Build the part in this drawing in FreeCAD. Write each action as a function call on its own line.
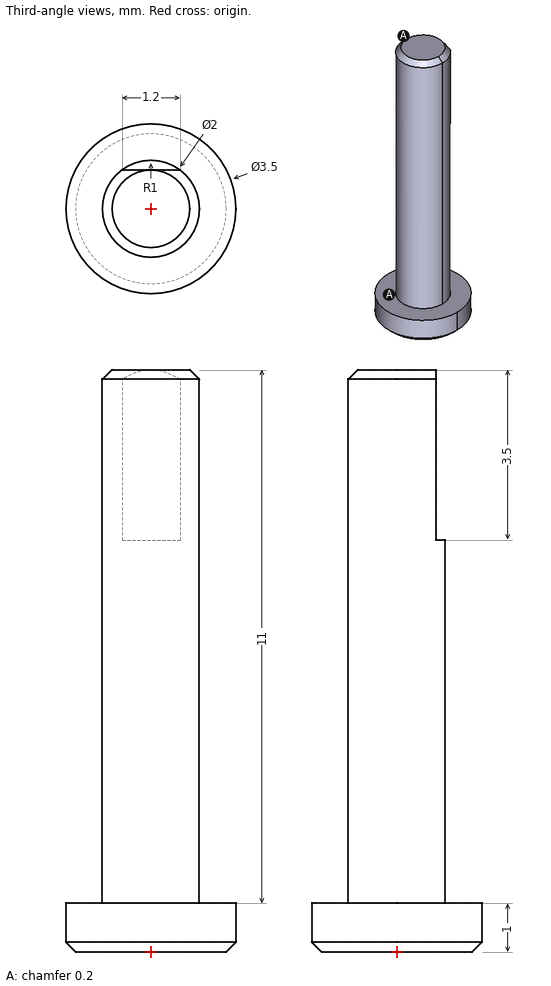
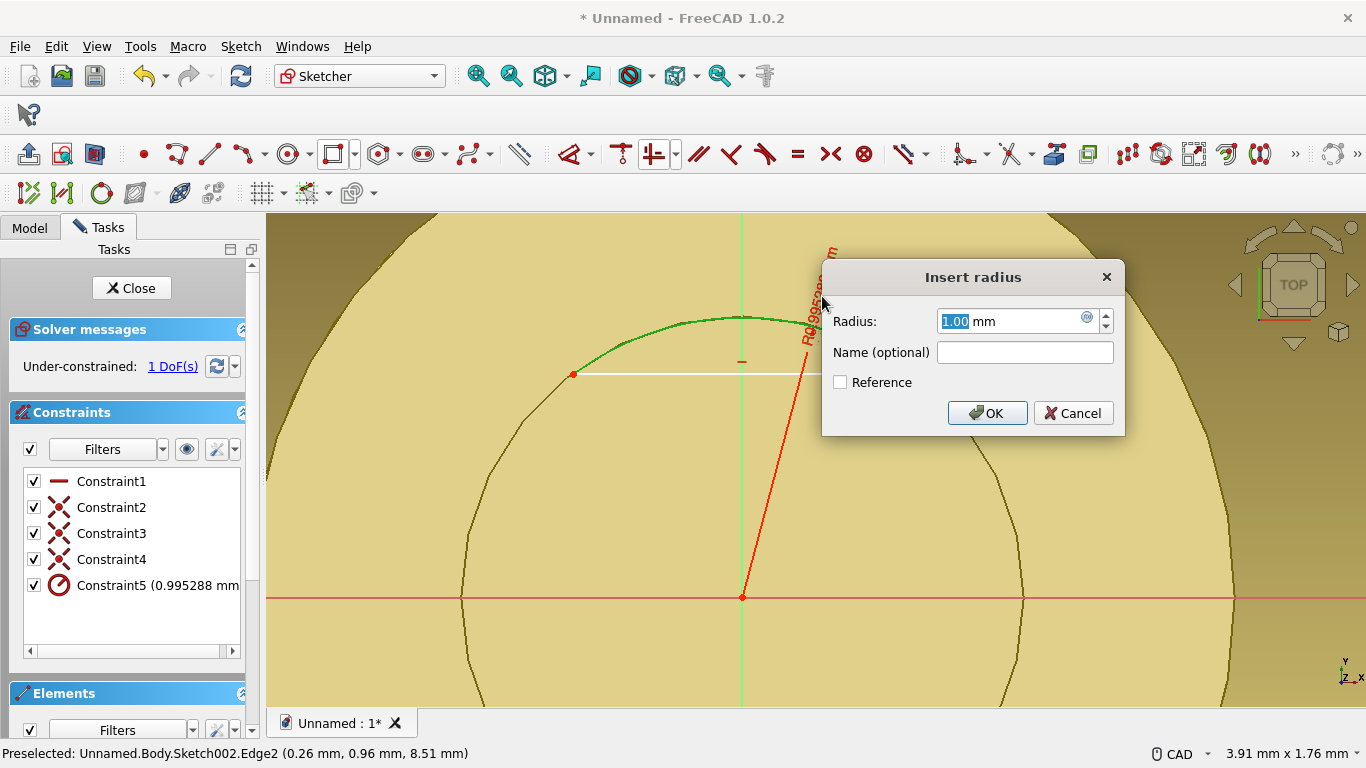
text(1)
key(Return)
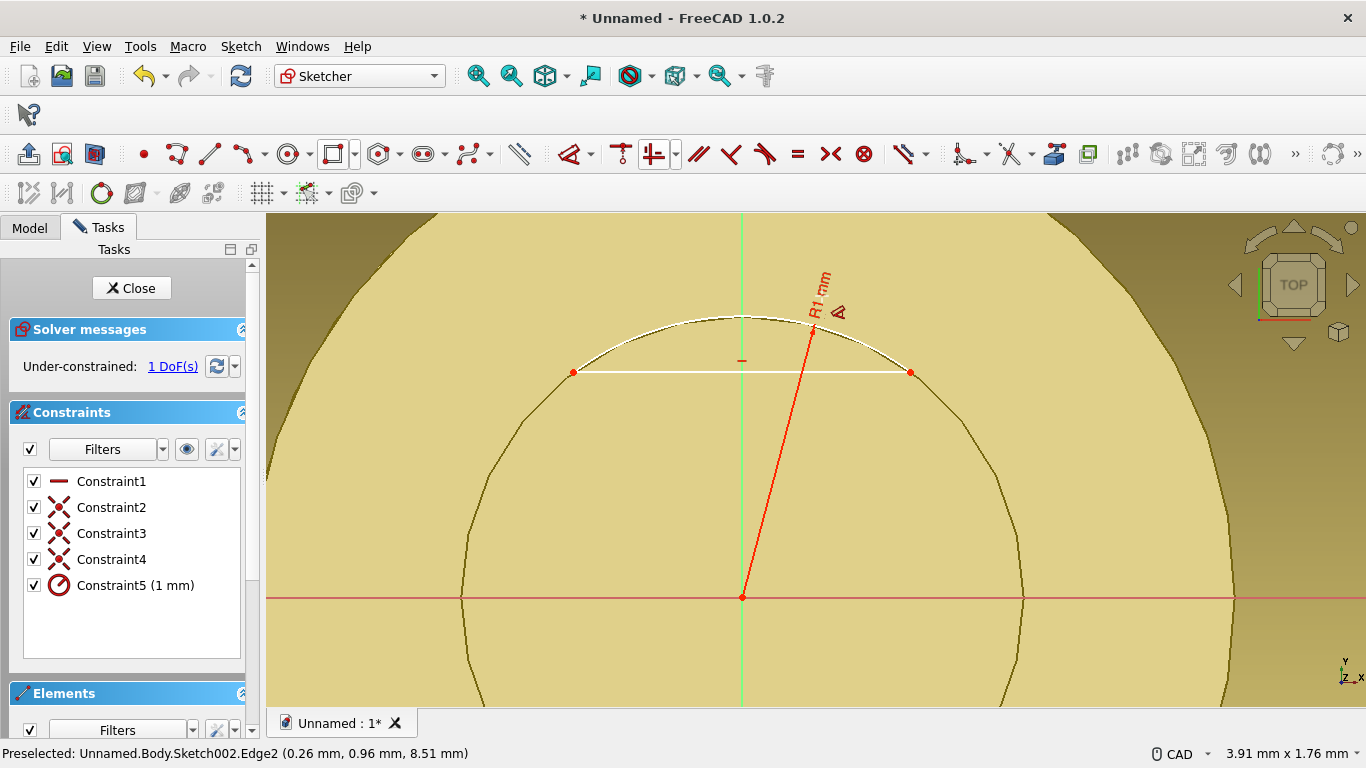
click(675, 372)
click(665, 406)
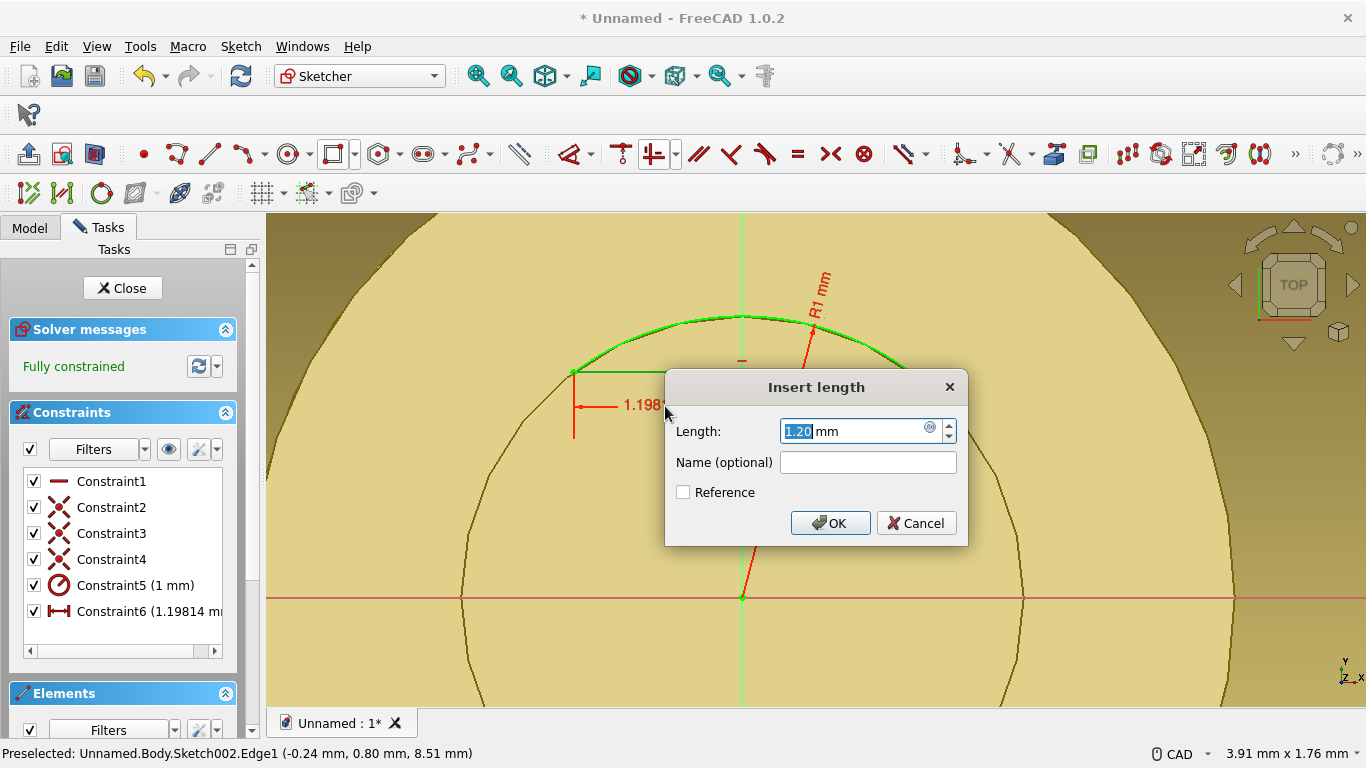
text(1.2)
key(Return)
key(Escape)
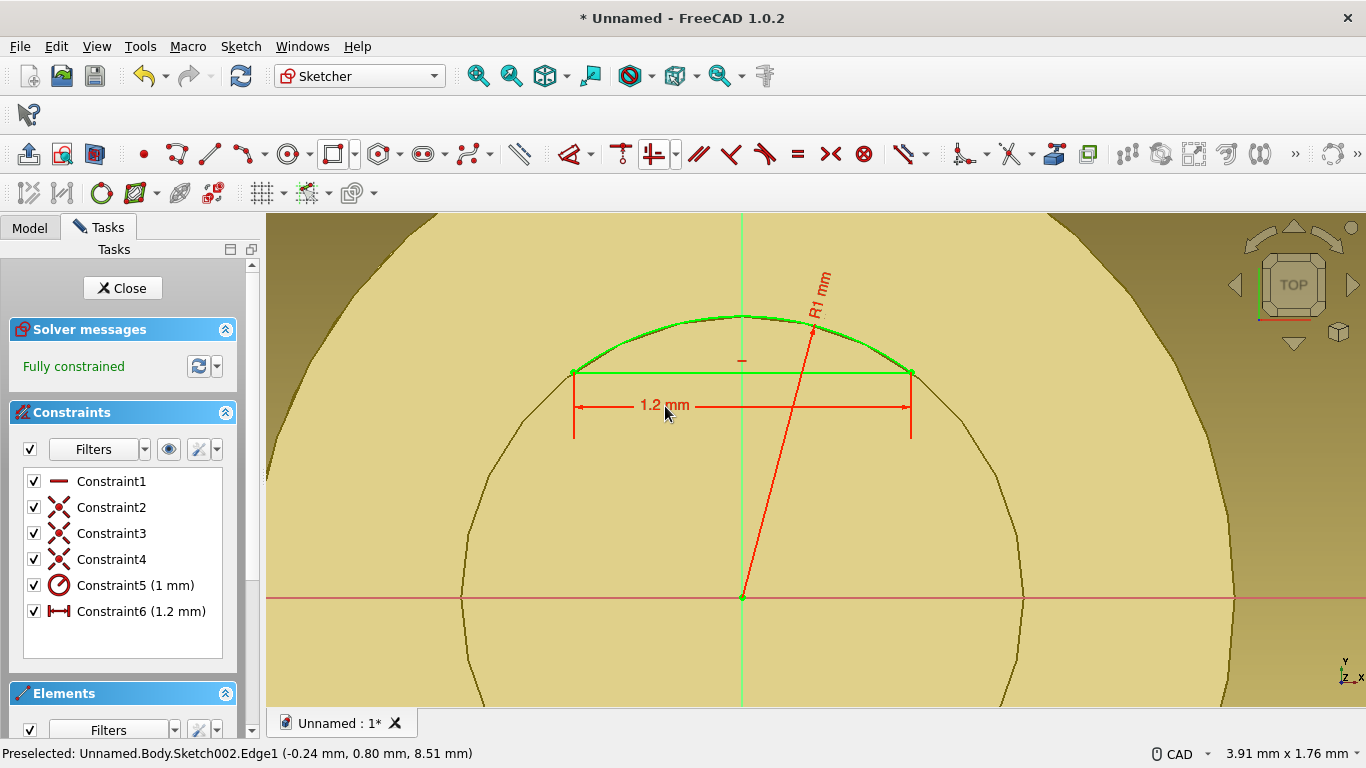
click(123, 288)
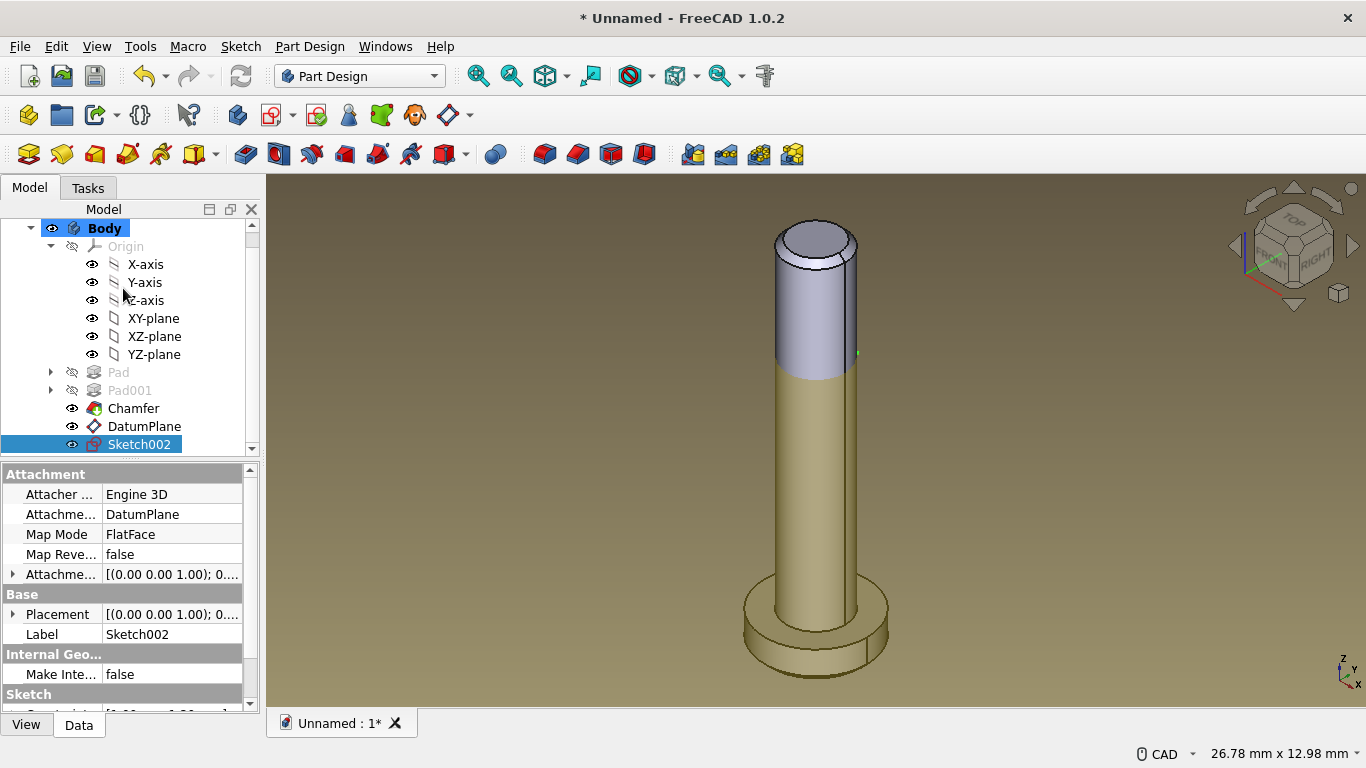
click(246, 154)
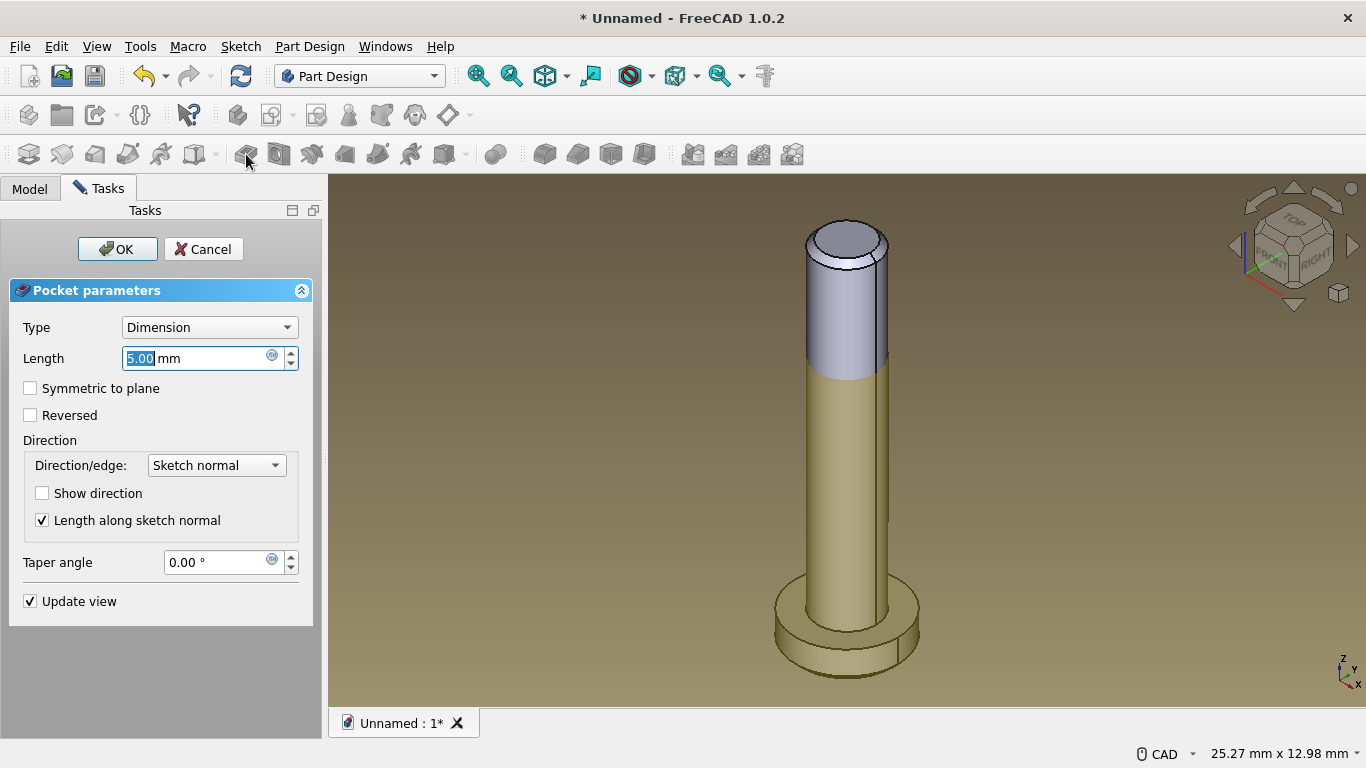
text(3.5)
key(Tab)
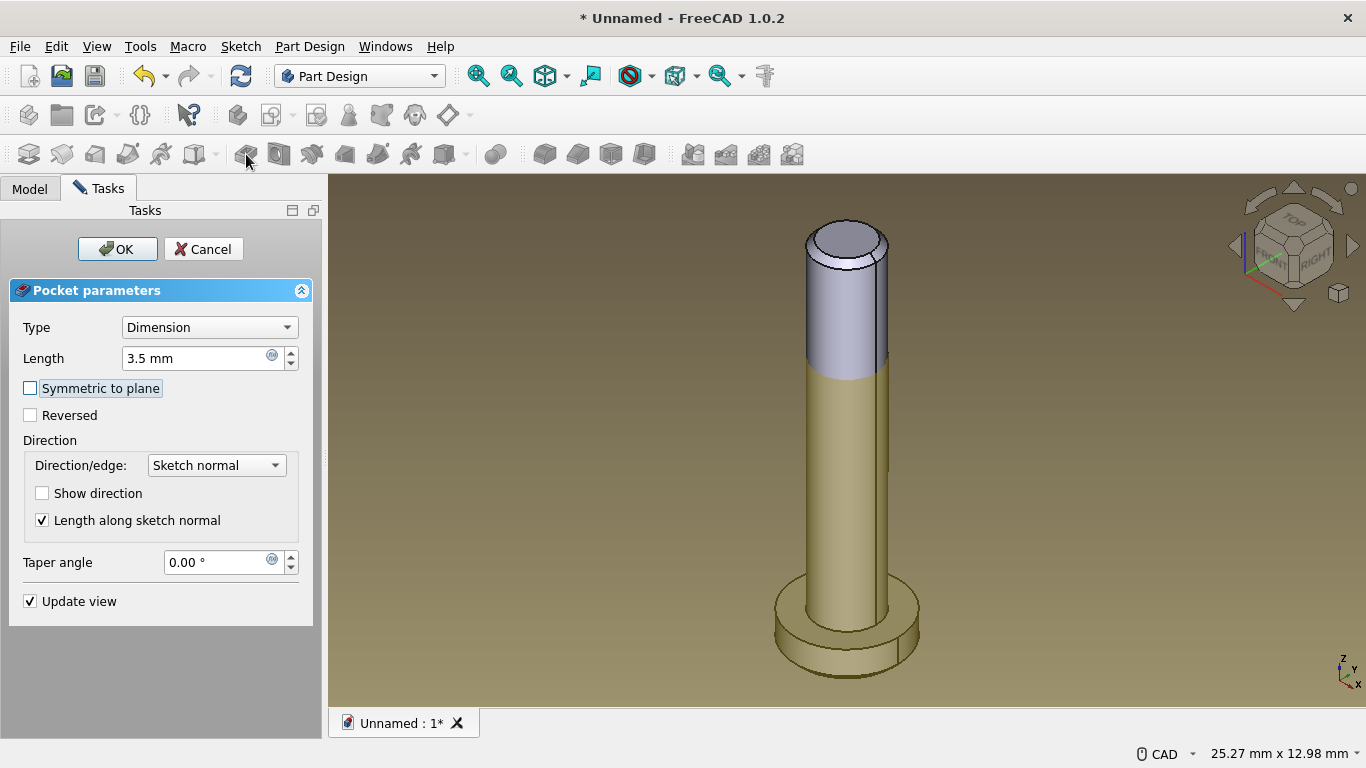
click(31, 415)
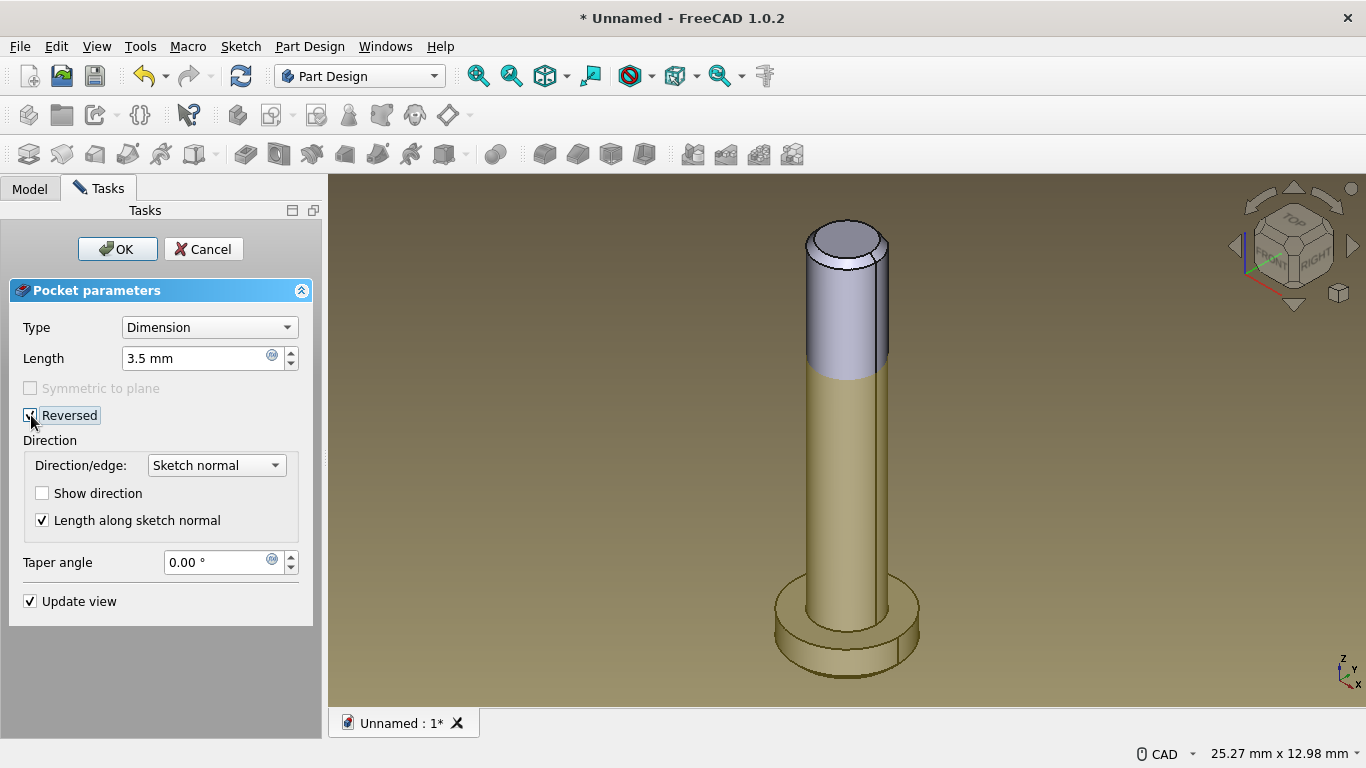
click(118, 249)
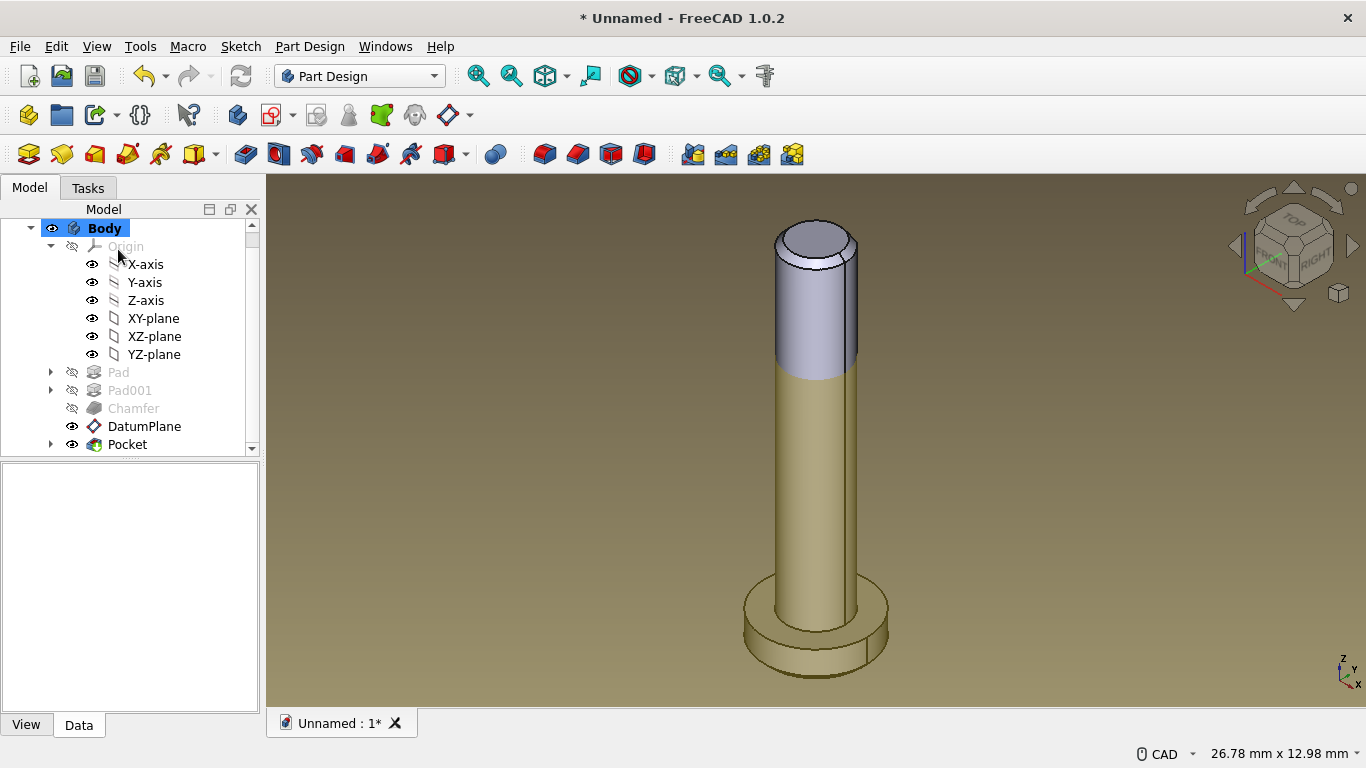
click(117, 426)
key(space)